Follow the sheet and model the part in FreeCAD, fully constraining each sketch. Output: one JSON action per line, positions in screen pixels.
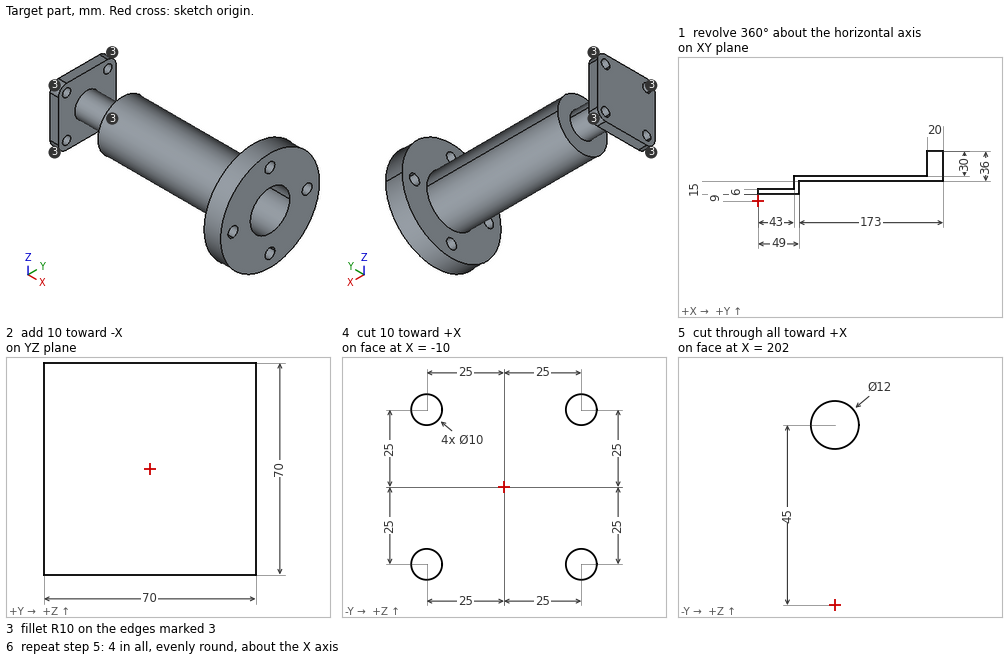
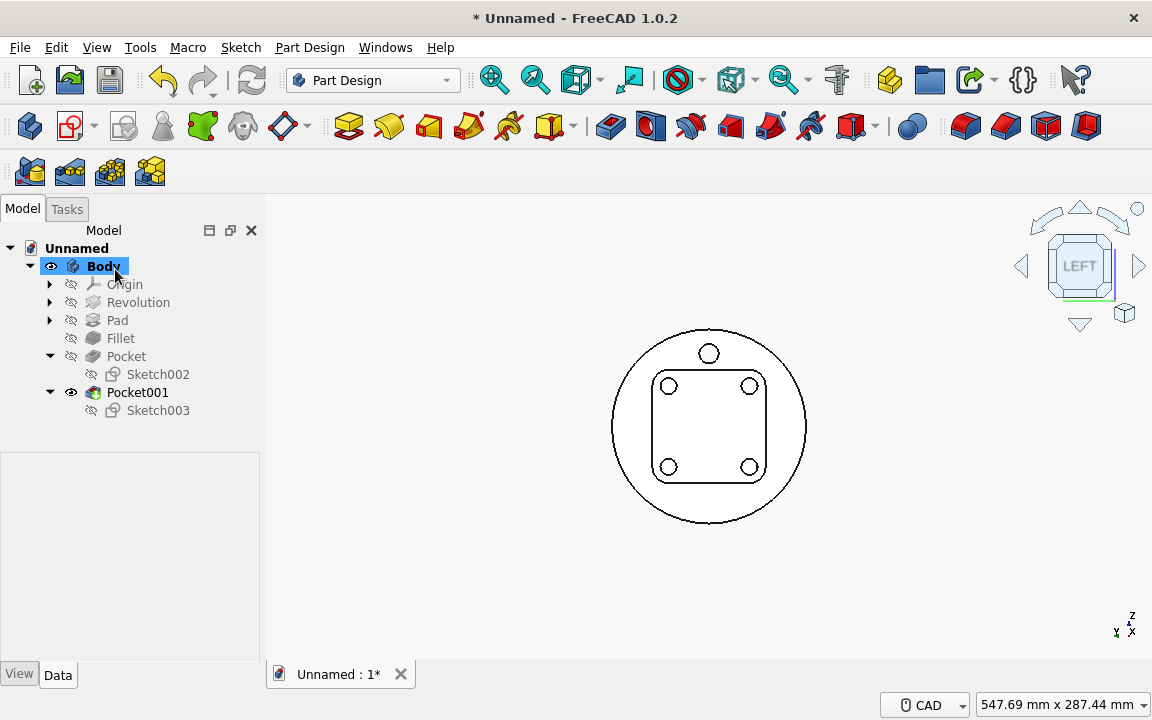
{"action": "left_click", "coordinate": [496, 80]}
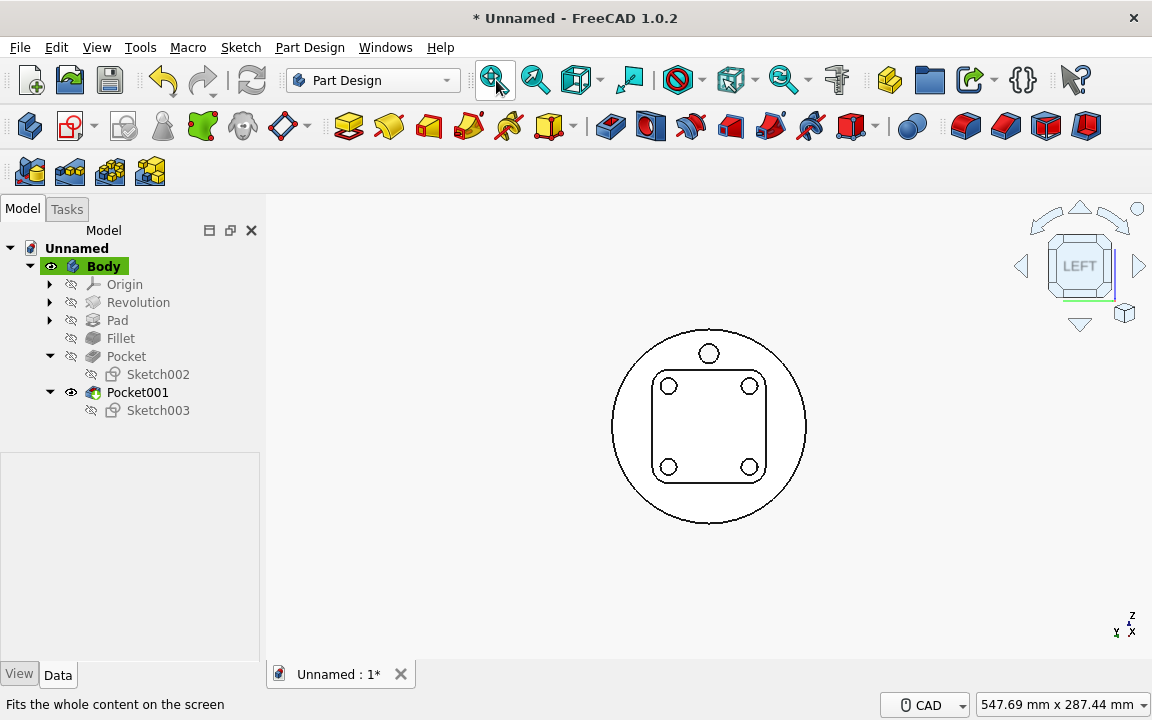
{"action": "left_click", "coordinate": [116, 392]}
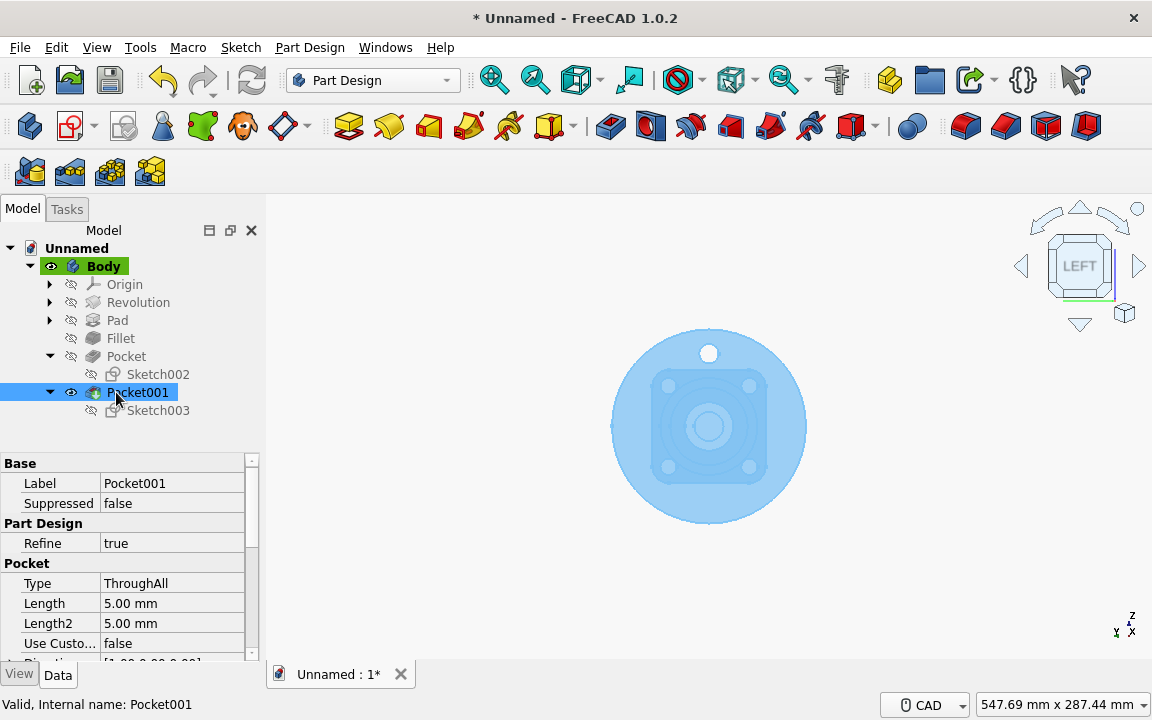
{"action": "left_click", "coordinate": [110, 172]}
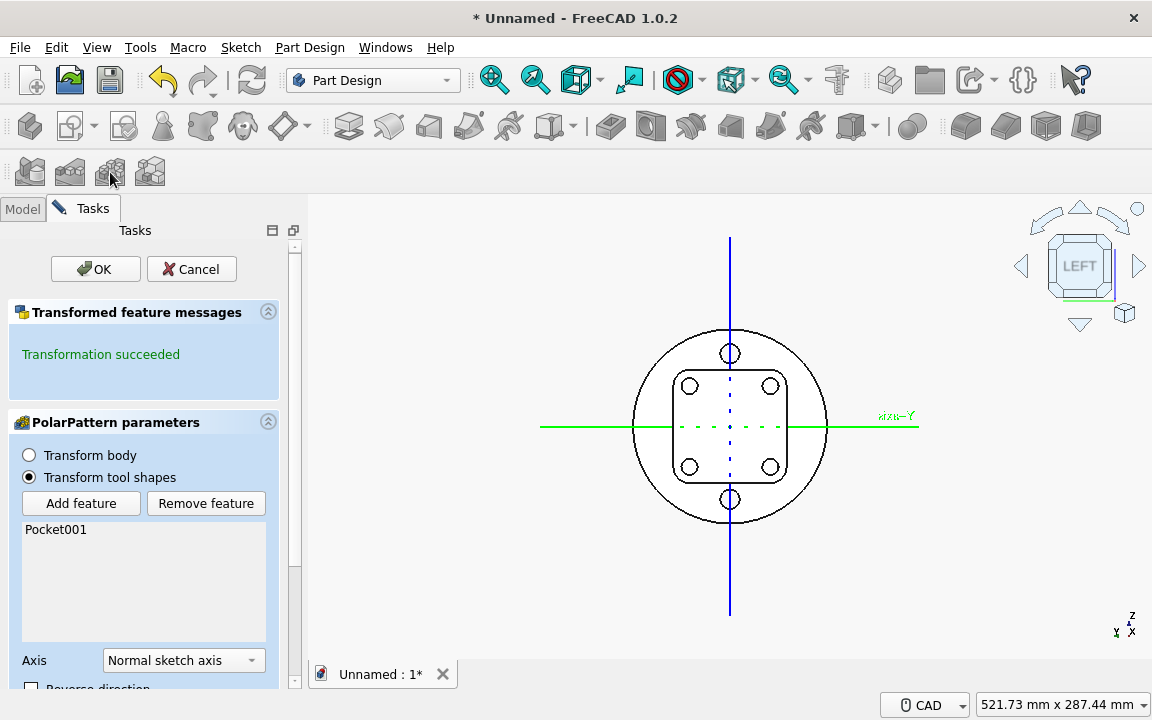
{"action": "left_click", "coordinate": [184, 660]}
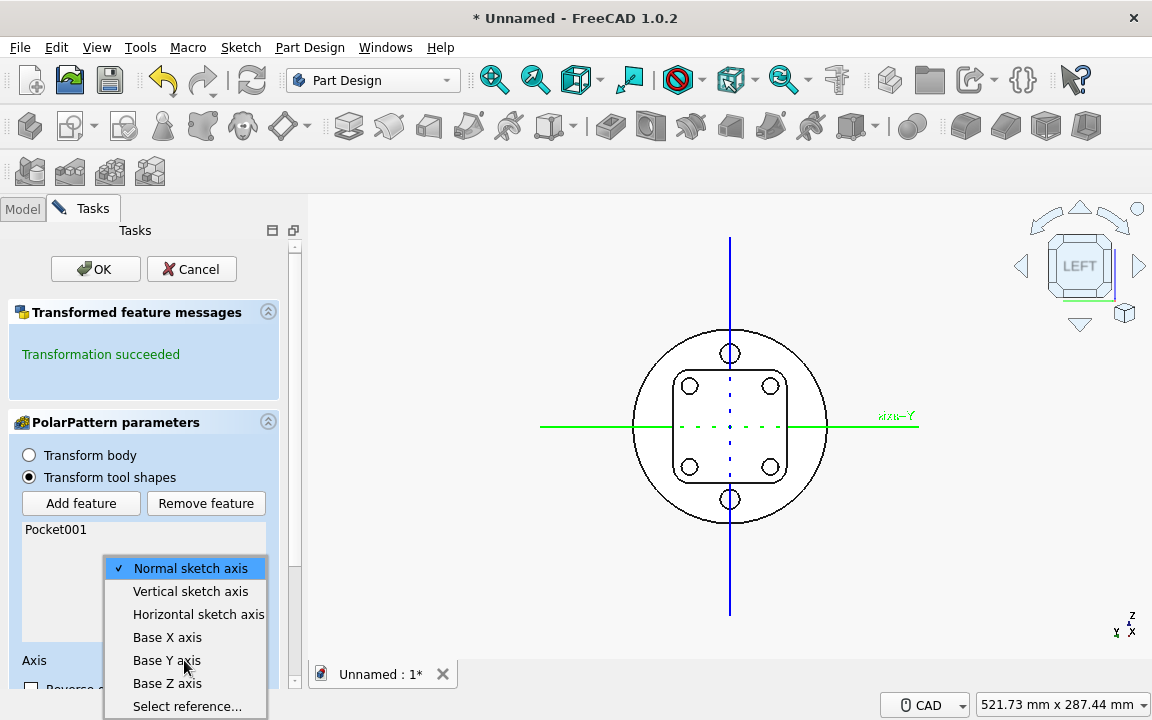
{"action": "left_click", "coordinate": [184, 638]}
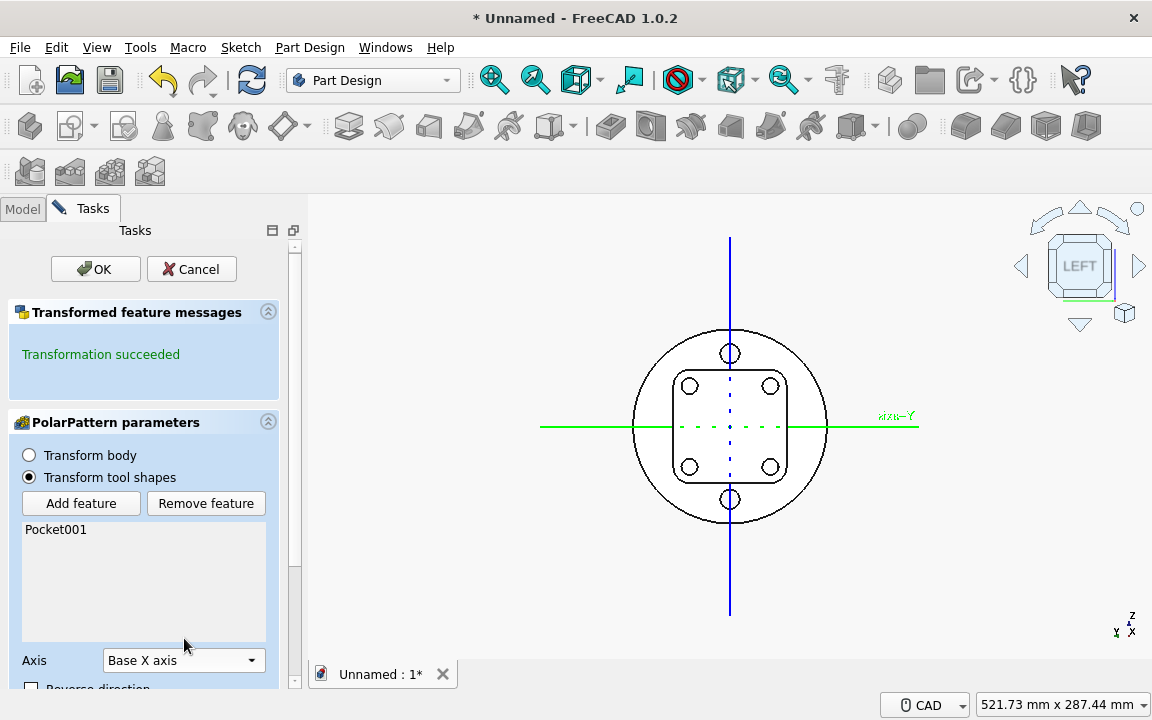
{"action": "scroll", "coordinate": [295, 464], "scroll_direction": "down", "scroll_amount": 3}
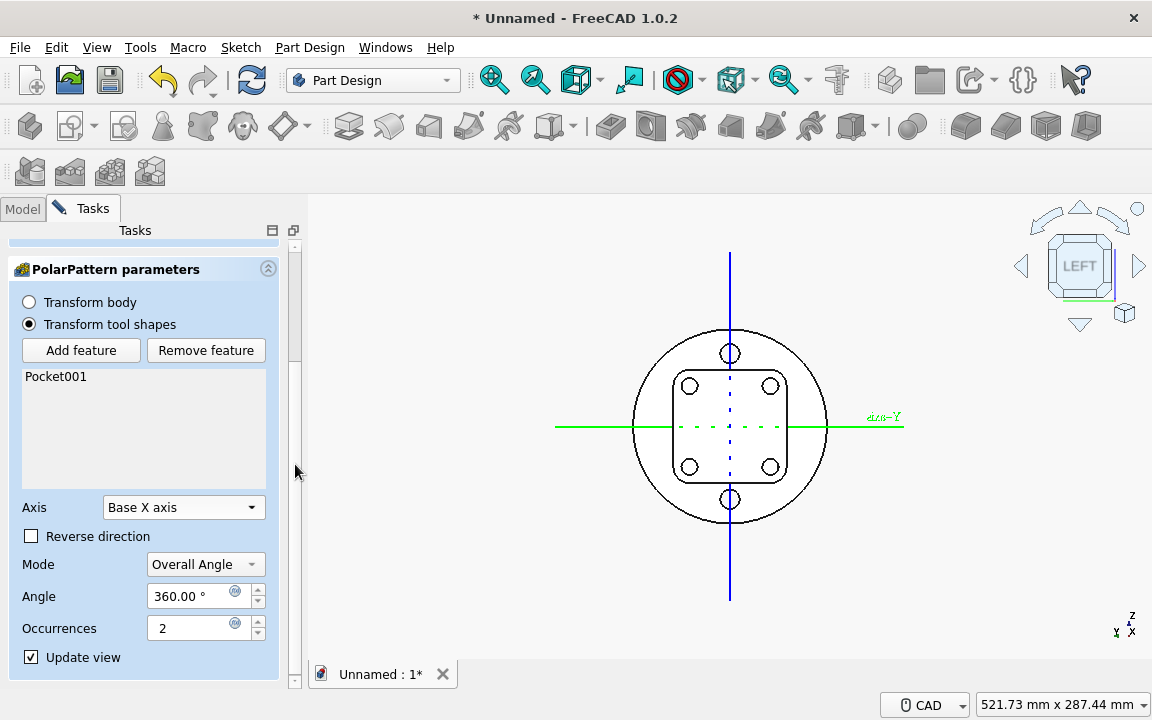
{"action": "triple_click", "coordinate": [198, 628]}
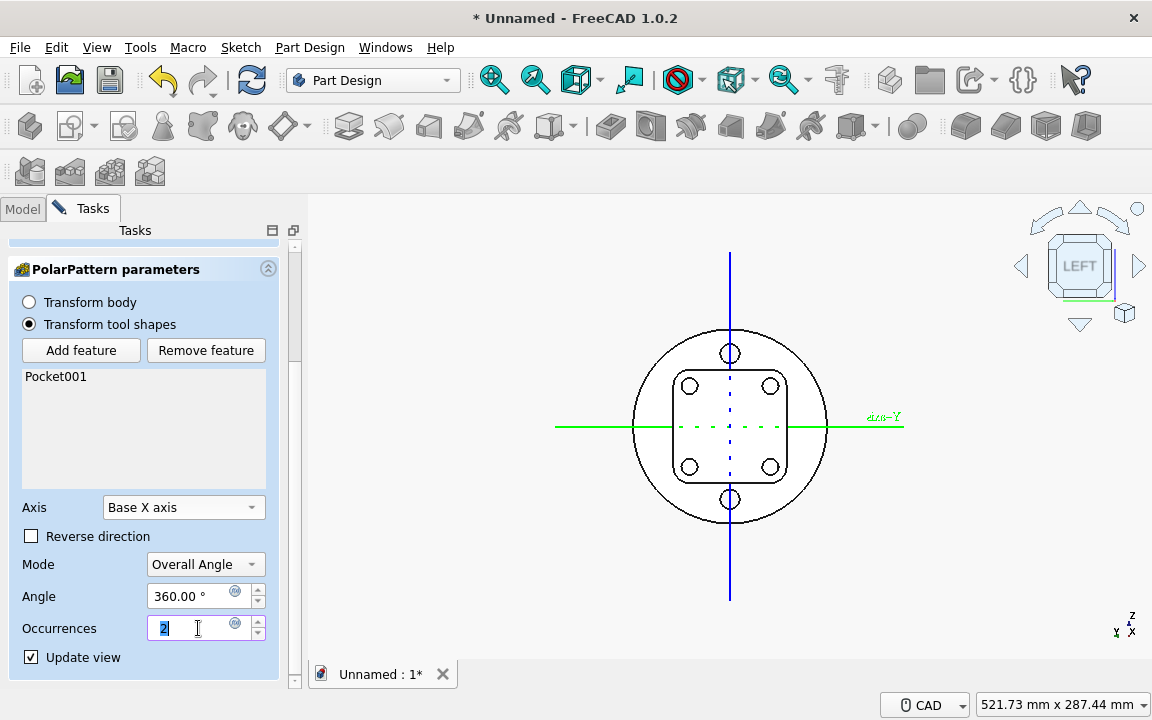
{"action": "type", "text": "4"}
{"action": "key", "text": "Tab"}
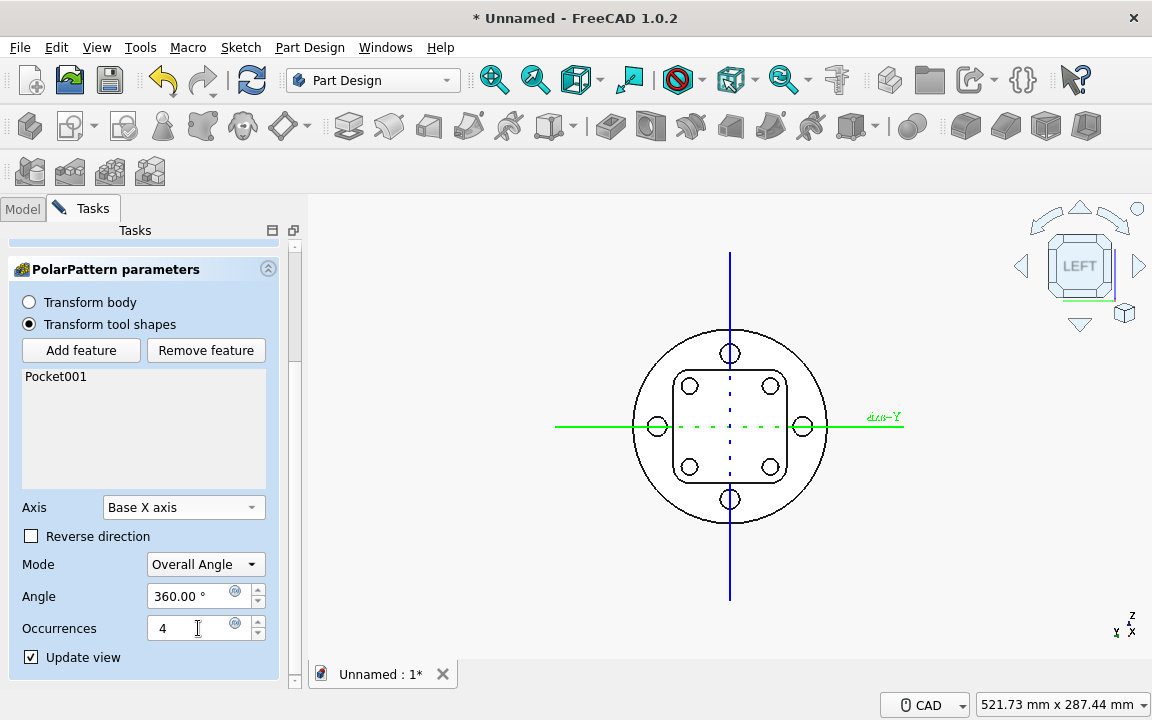
{"action": "scroll", "coordinate": [295, 464], "scroll_direction": "up", "scroll_amount": 4}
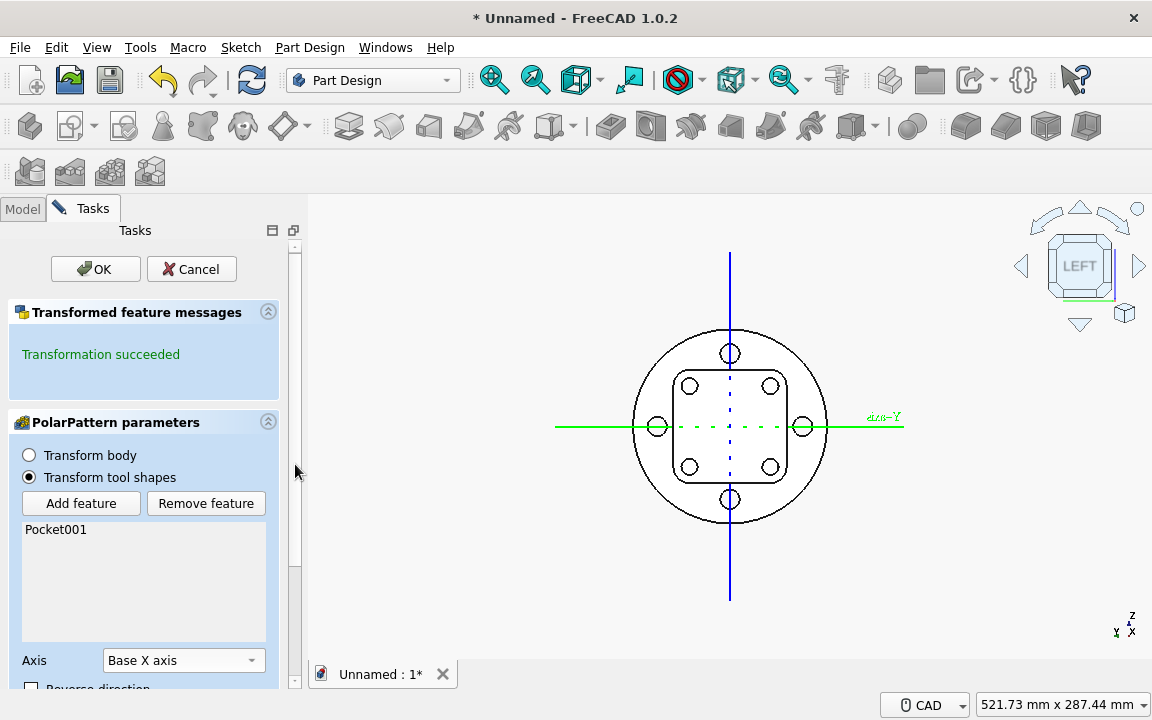
{"action": "left_click", "coordinate": [96, 269]}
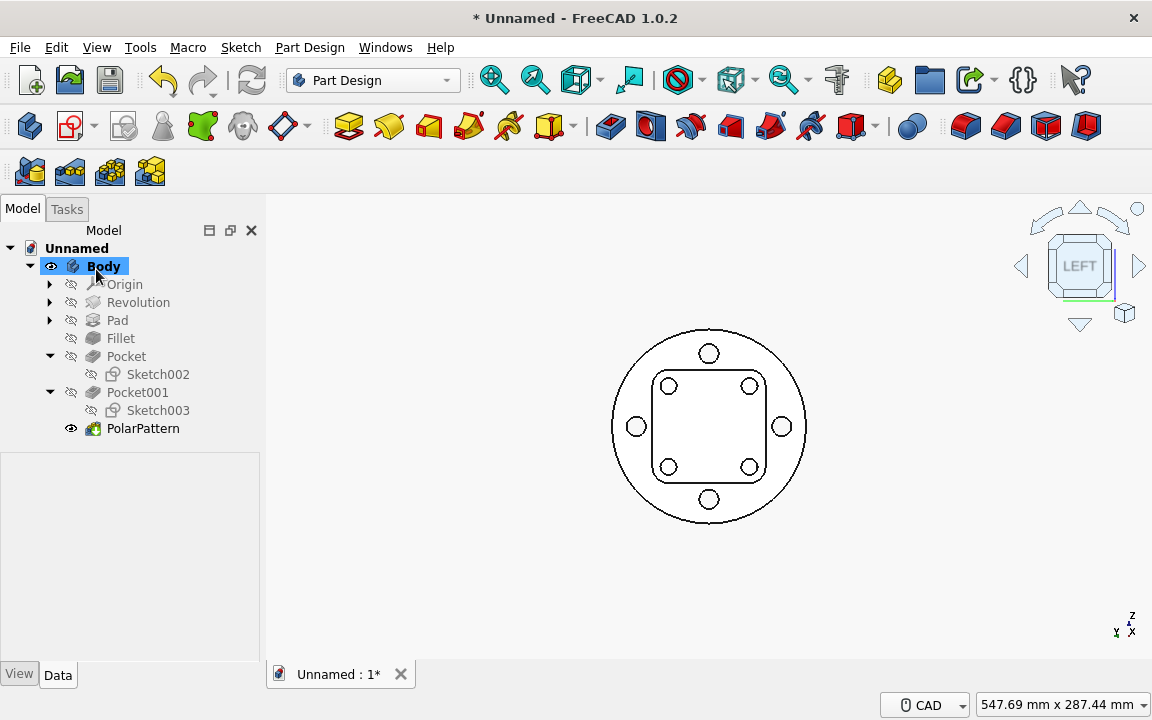
{"action": "key", "text": "0"}